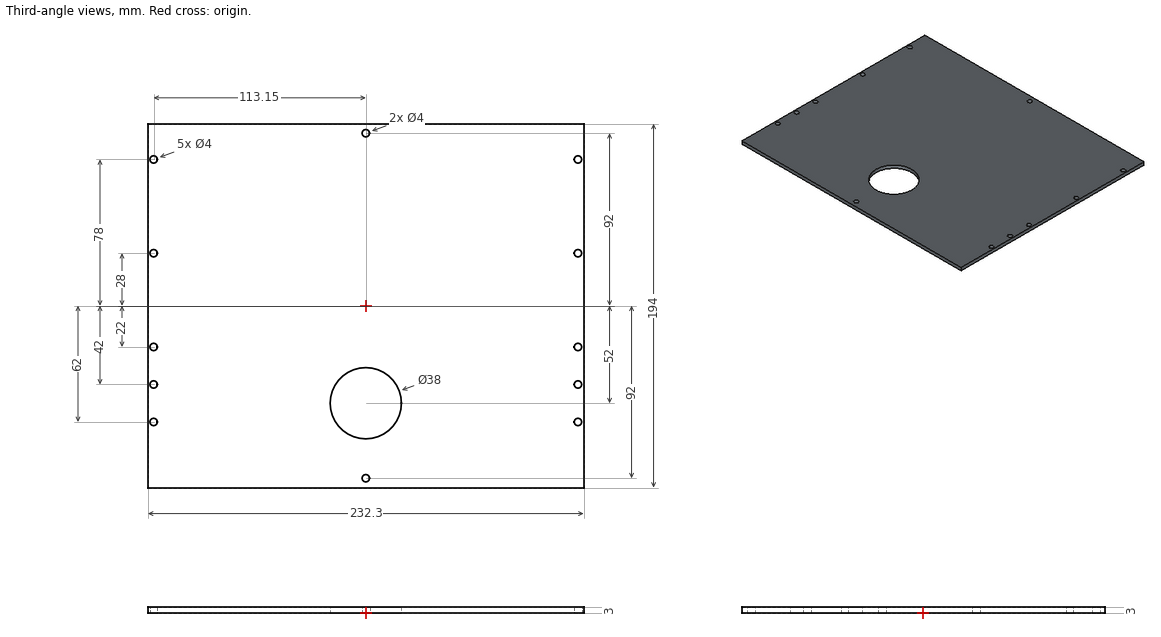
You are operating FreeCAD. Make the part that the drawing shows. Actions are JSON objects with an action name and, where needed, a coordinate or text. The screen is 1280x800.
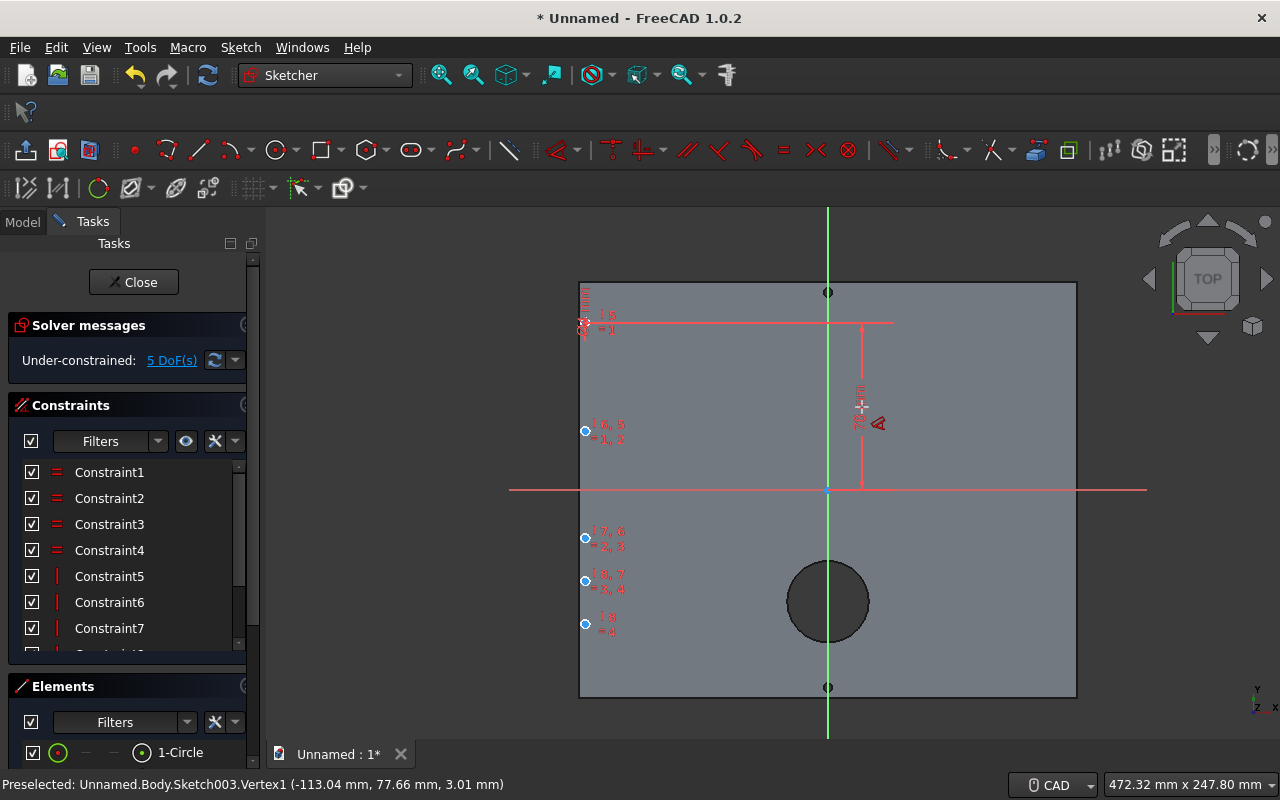
{"action": "left_click", "coordinate": [585, 431]}
{"action": "left_click", "coordinate": [862, 461]}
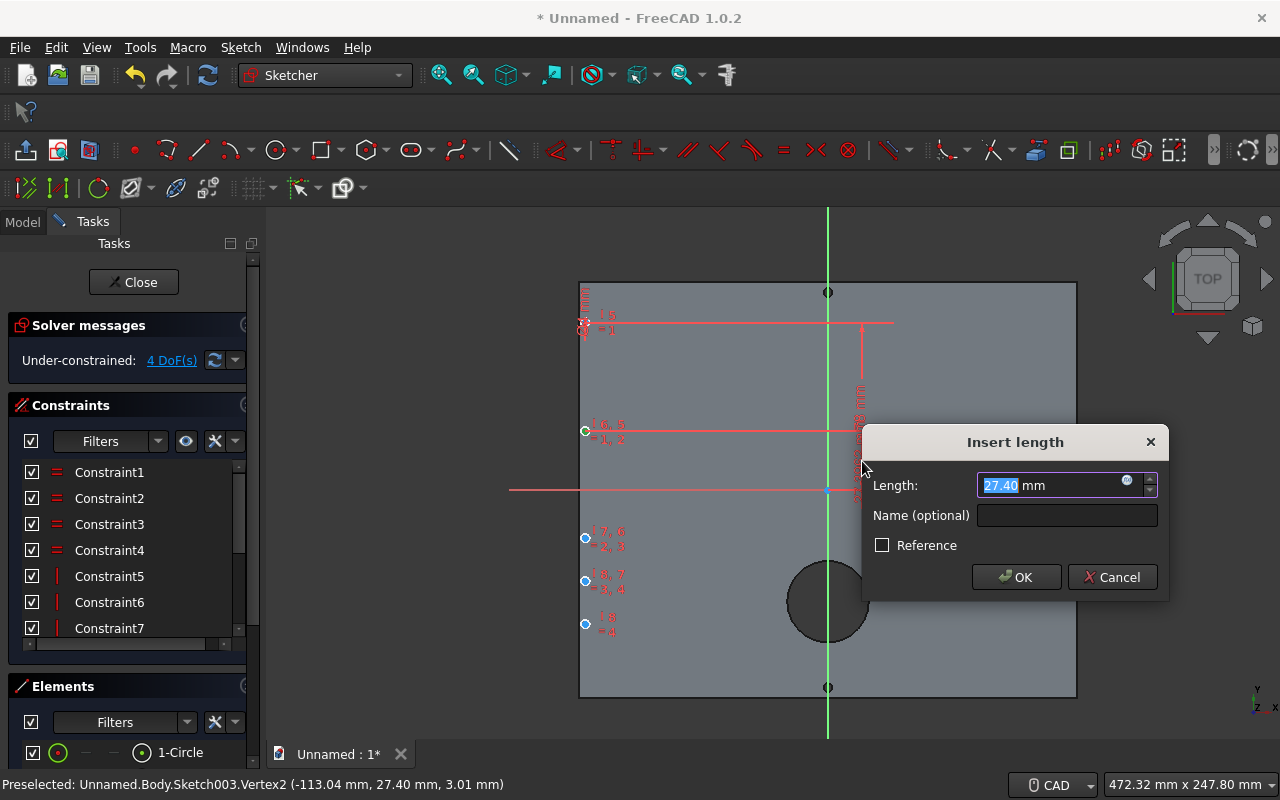
{"action": "type", "text": "28"}
{"action": "key", "text": "Return"}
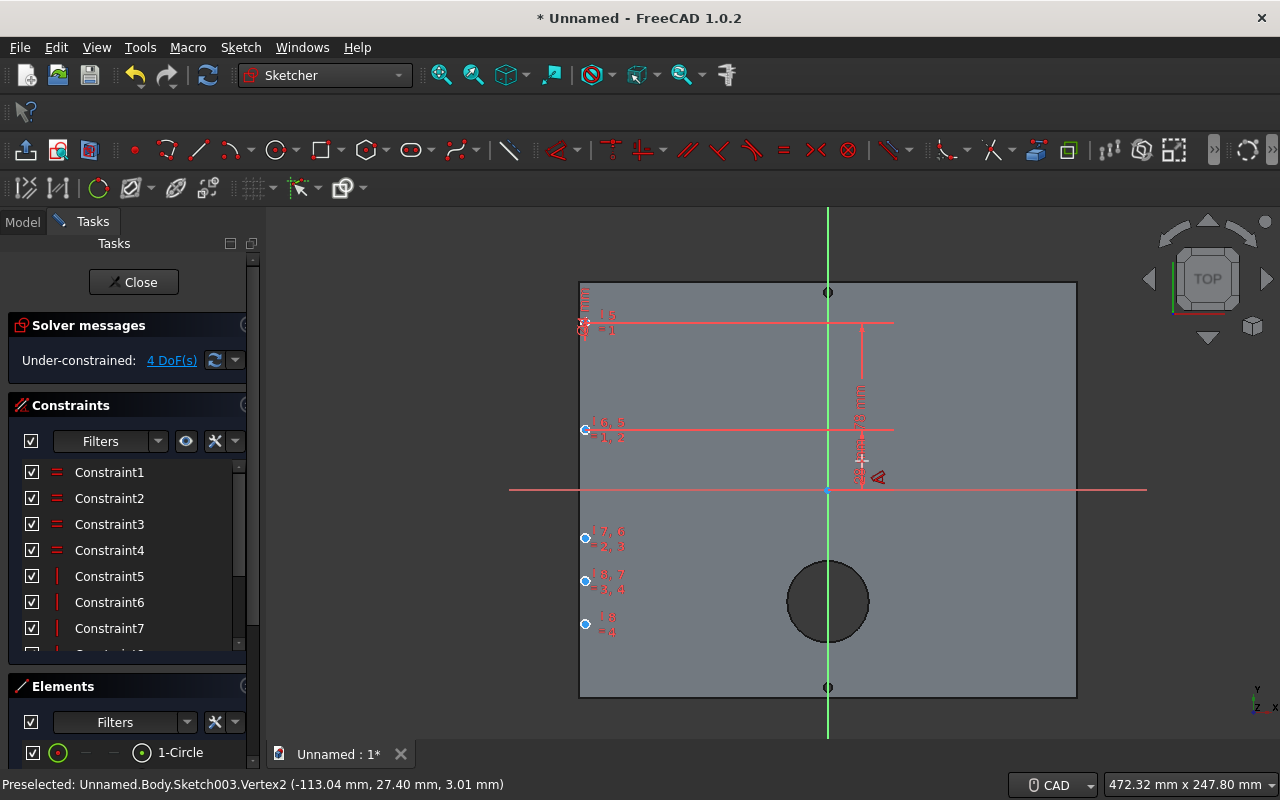
{"action": "left_click", "coordinate": [585, 538]}
{"action": "left_click", "coordinate": [862, 514]}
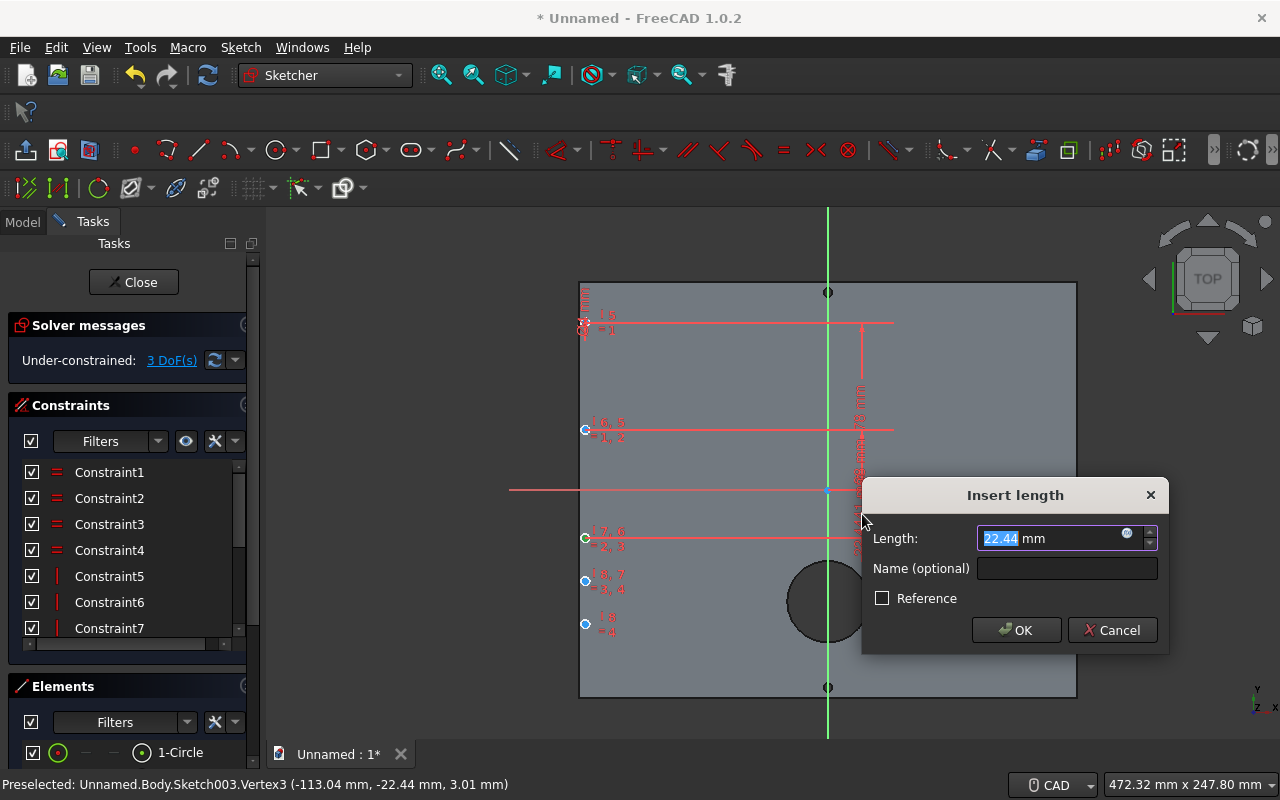
{"action": "type", "text": "22"}
{"action": "key", "text": "Return"}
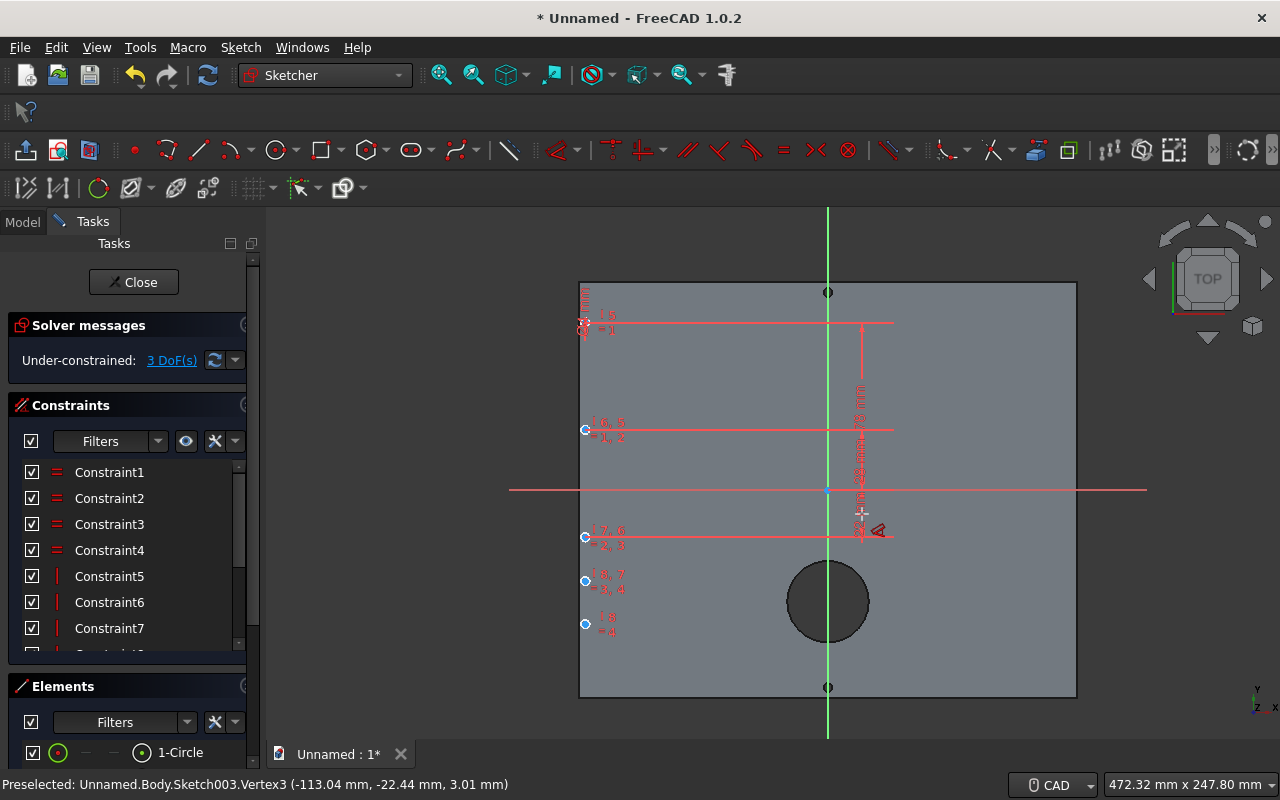
{"action": "left_click", "coordinate": [585, 581]}
{"action": "left_click", "coordinate": [862, 536]}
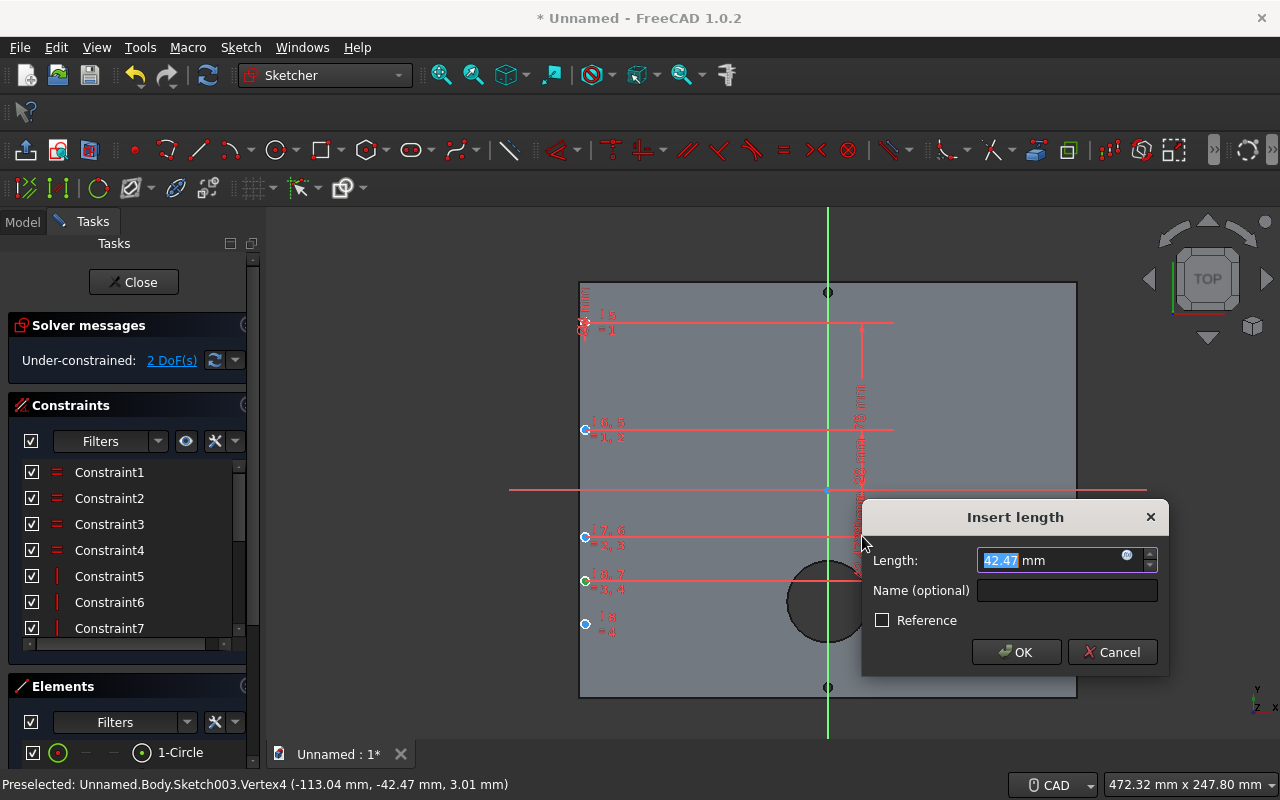
{"action": "type", "text": "42"}
{"action": "key", "text": "Return"}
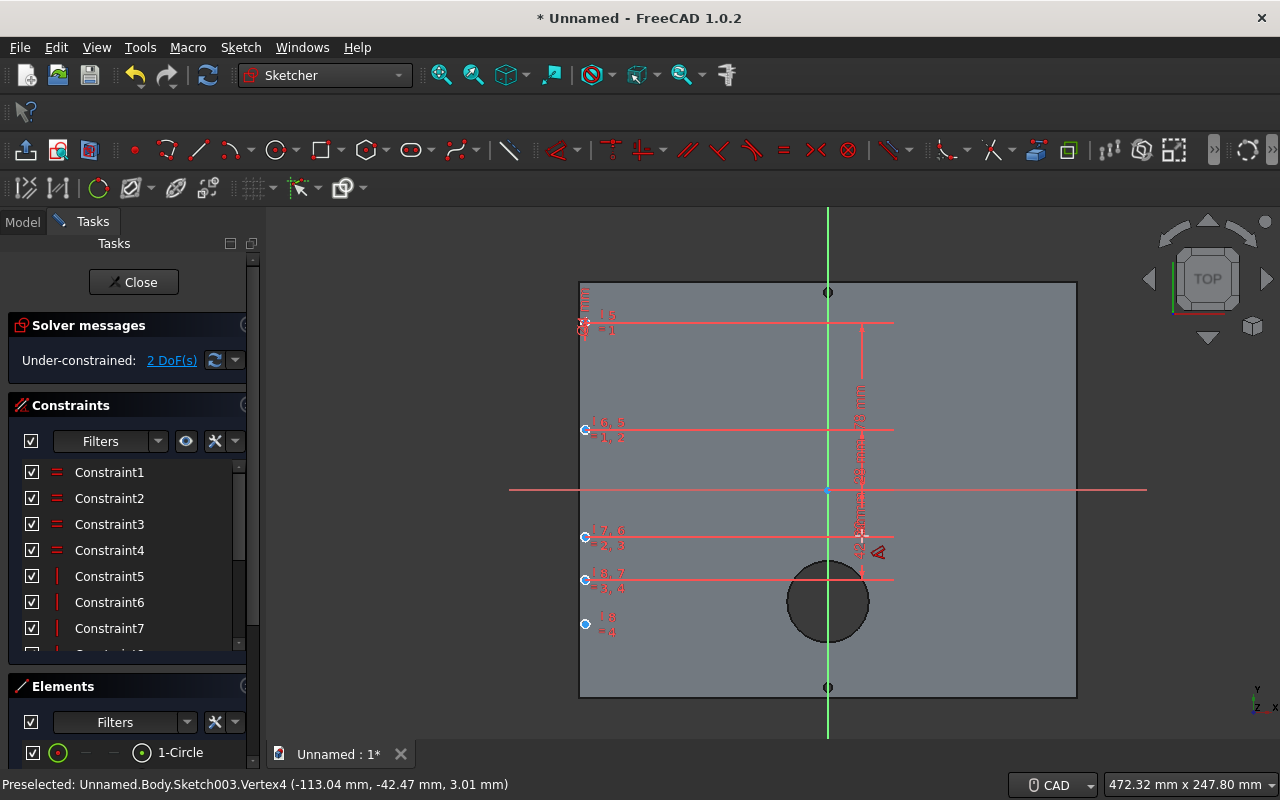
{"action": "left_click", "coordinate": [585, 624]}
{"action": "left_click", "coordinate": [862, 557]}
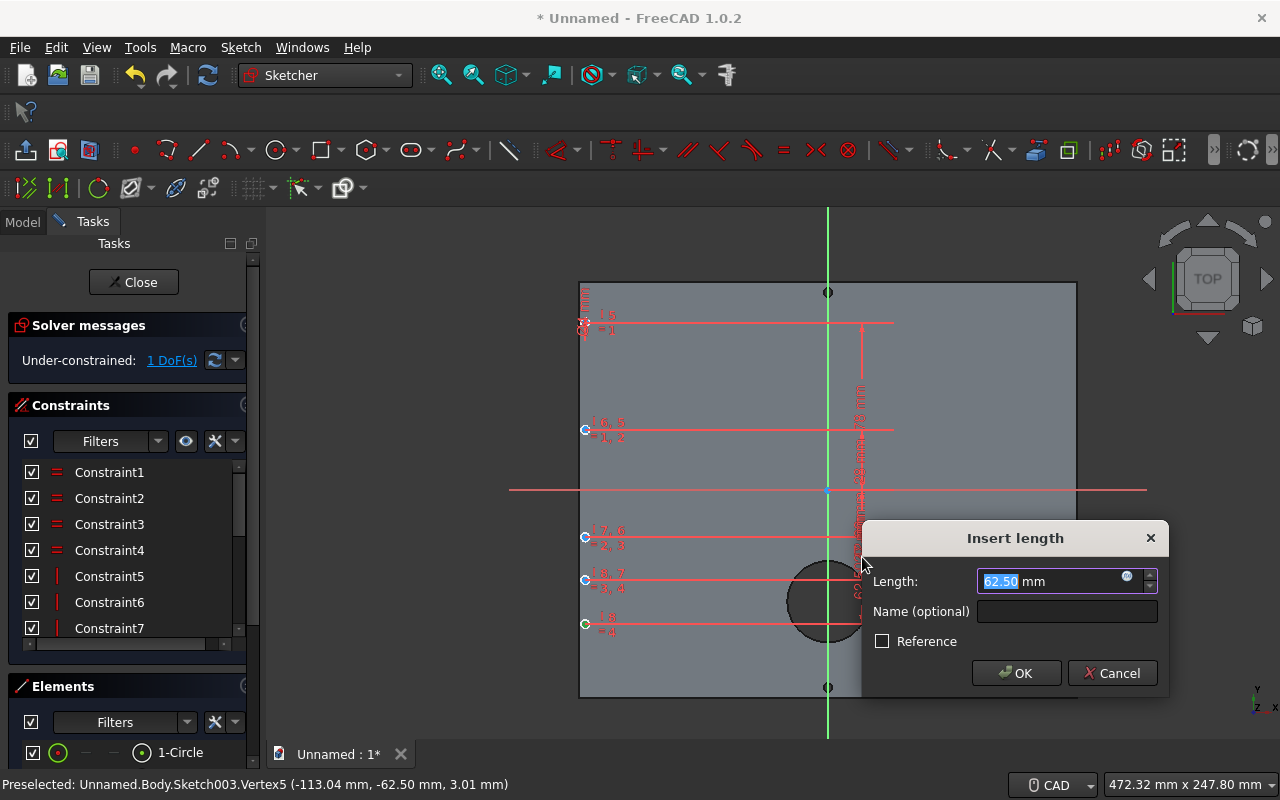
{"action": "type", "text": "62"}
{"action": "key", "text": "Return"}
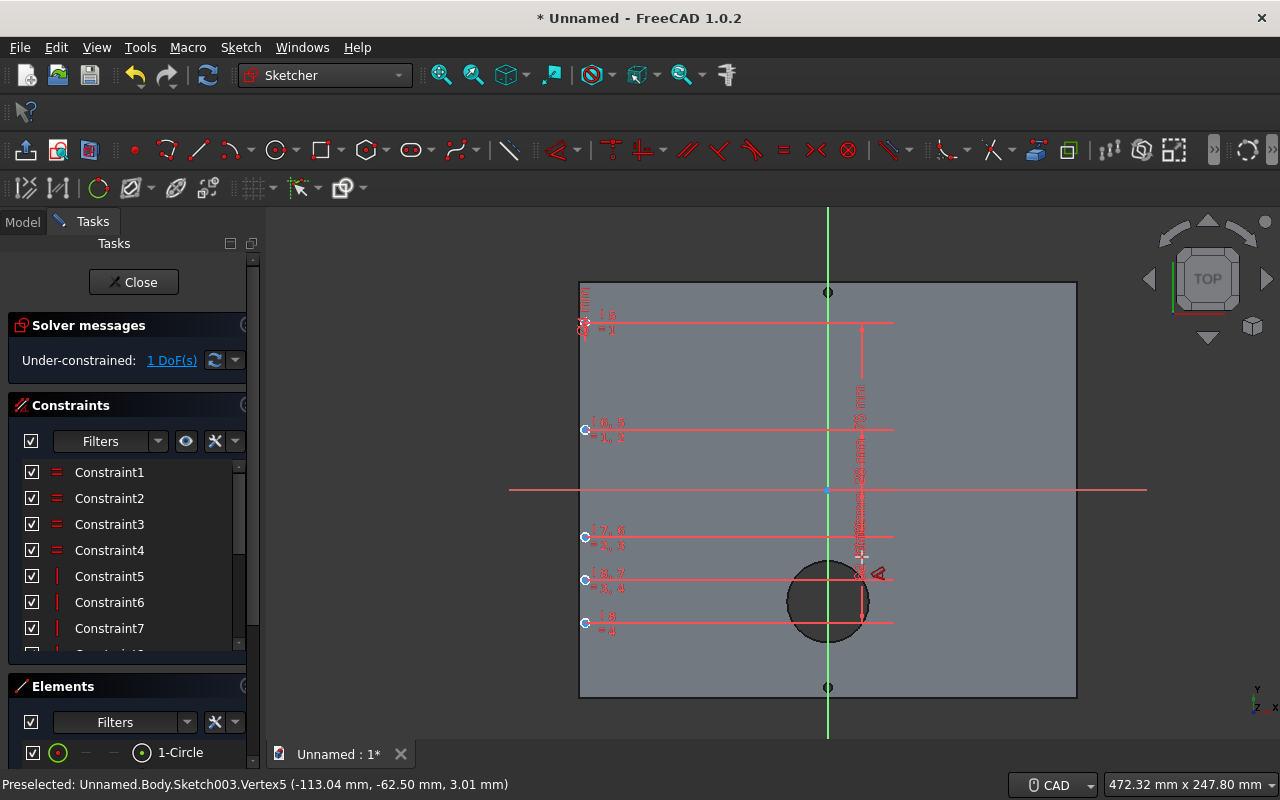
{"action": "left_click", "coordinate": [585, 323]}
{"action": "left_click", "coordinate": [707, 289]}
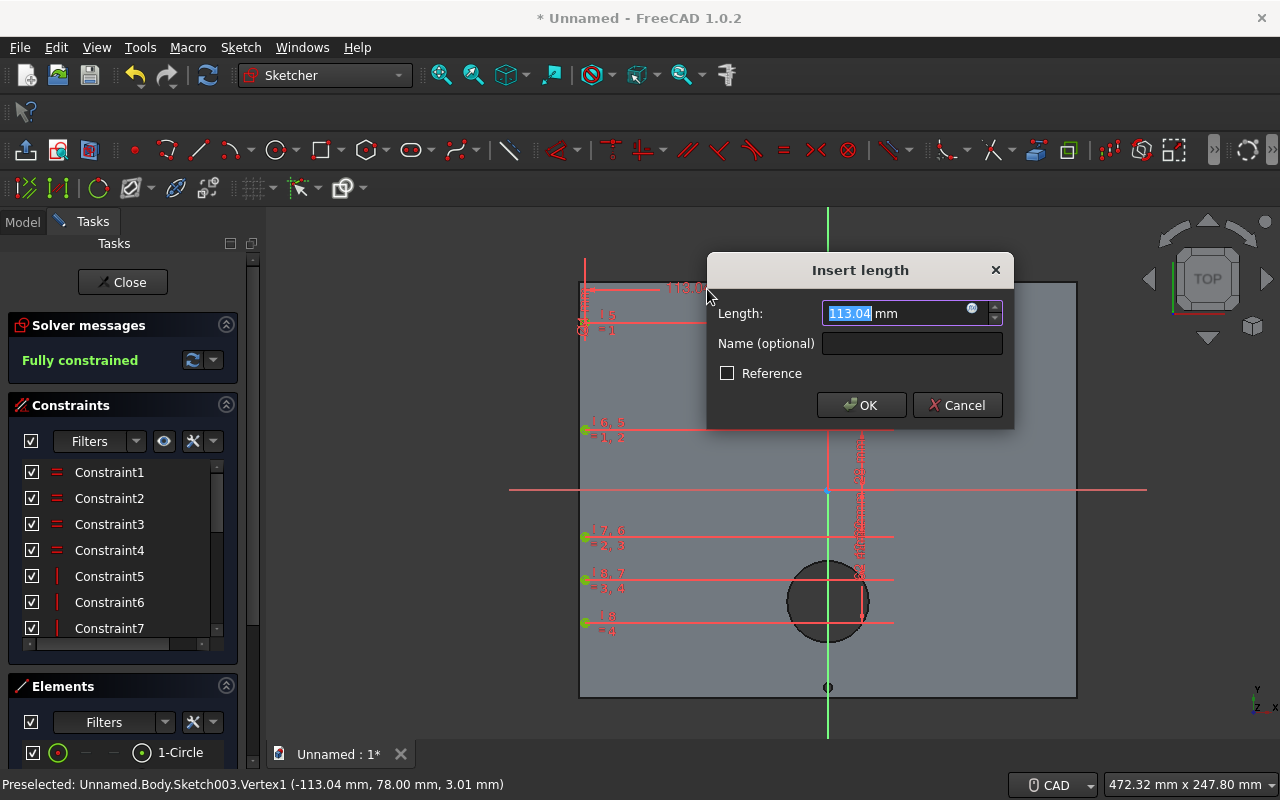
{"action": "type", "text": "113.15"}
{"action": "key", "text": "Return"}
{"action": "key", "text": "Escape"}